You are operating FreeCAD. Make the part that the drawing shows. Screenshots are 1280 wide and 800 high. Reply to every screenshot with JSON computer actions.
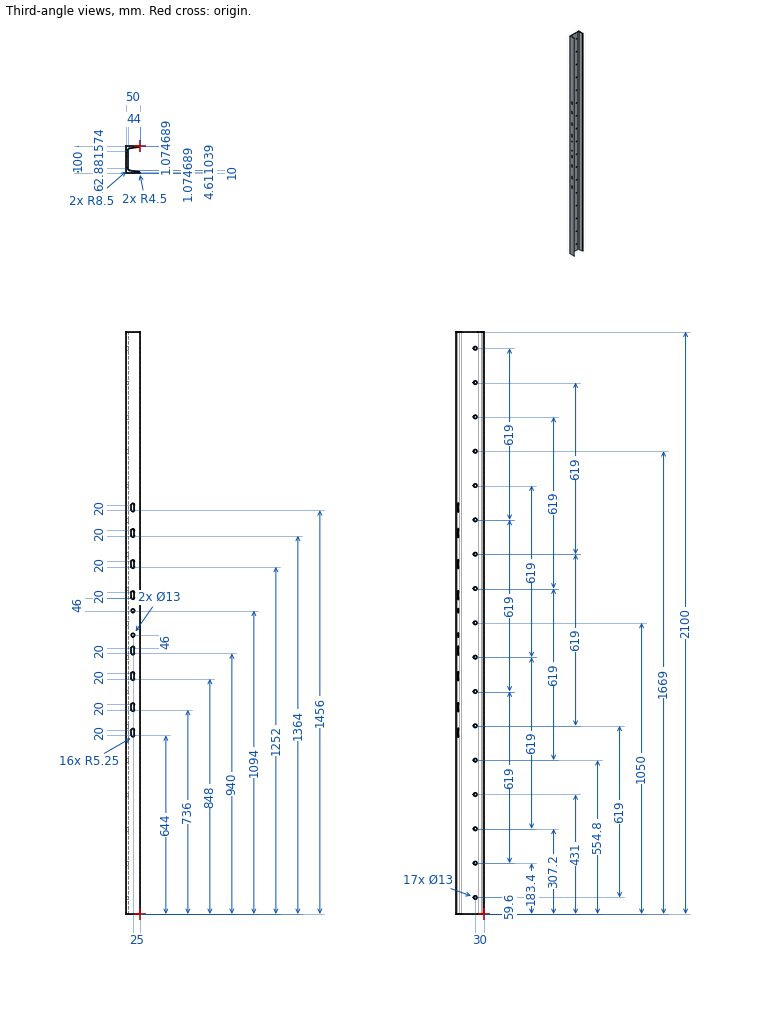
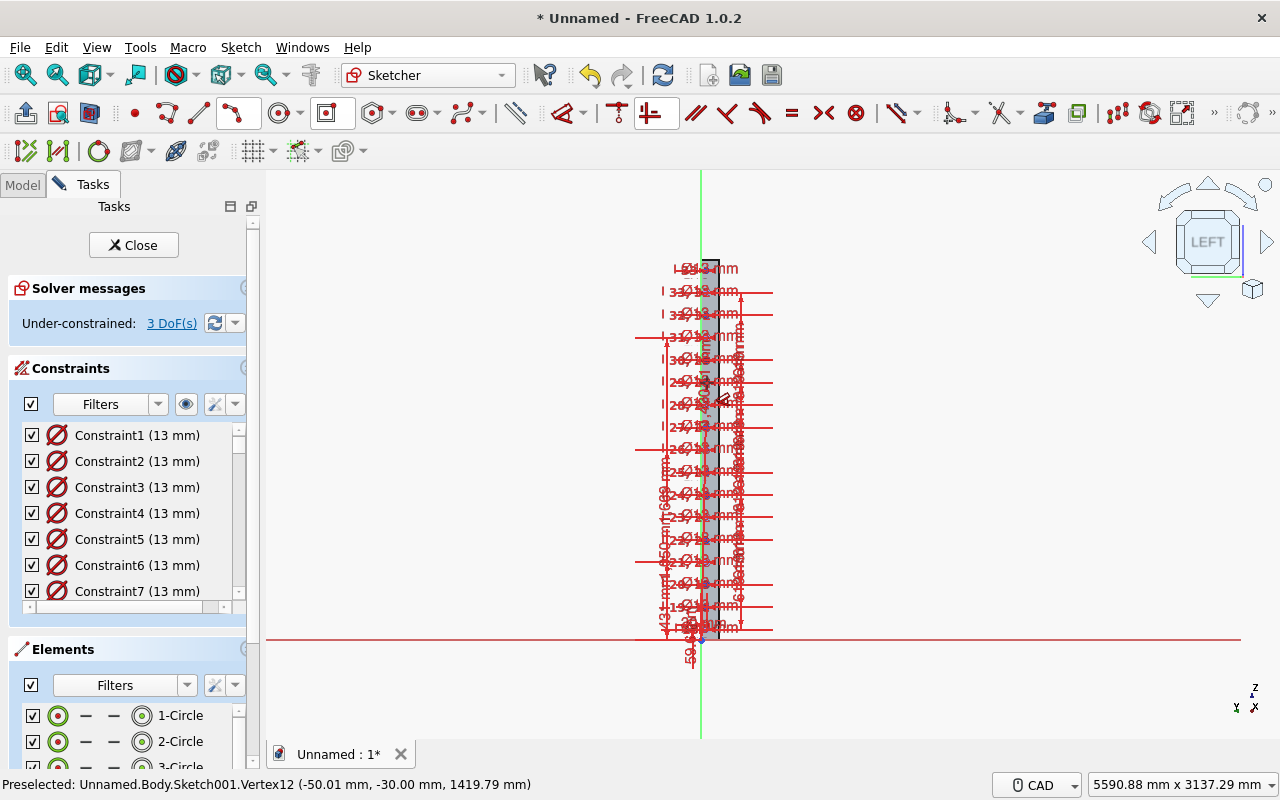
{"action": "left_click", "coordinate": [707, 271]}
{"action": "left_click", "coordinate": [741, 327]}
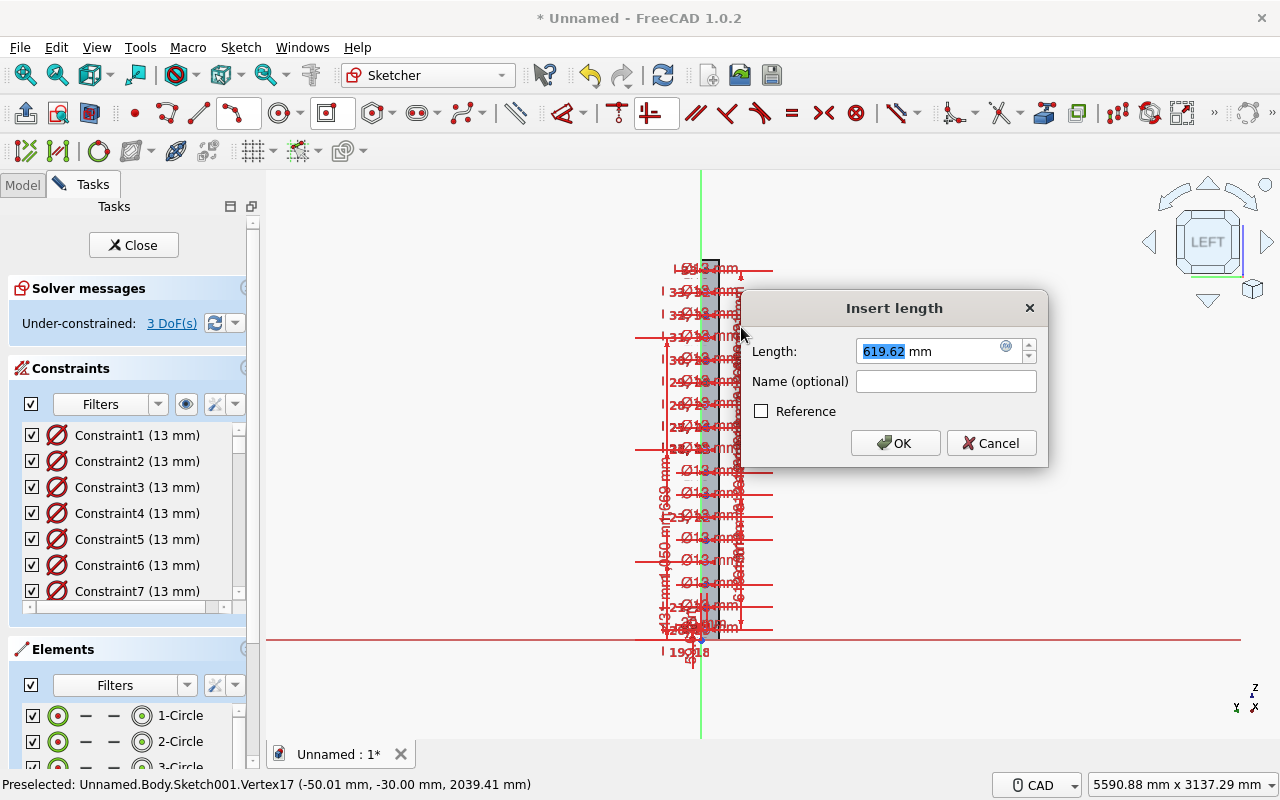
{"action": "type", "text": "619"}
{"action": "key", "text": "Return"}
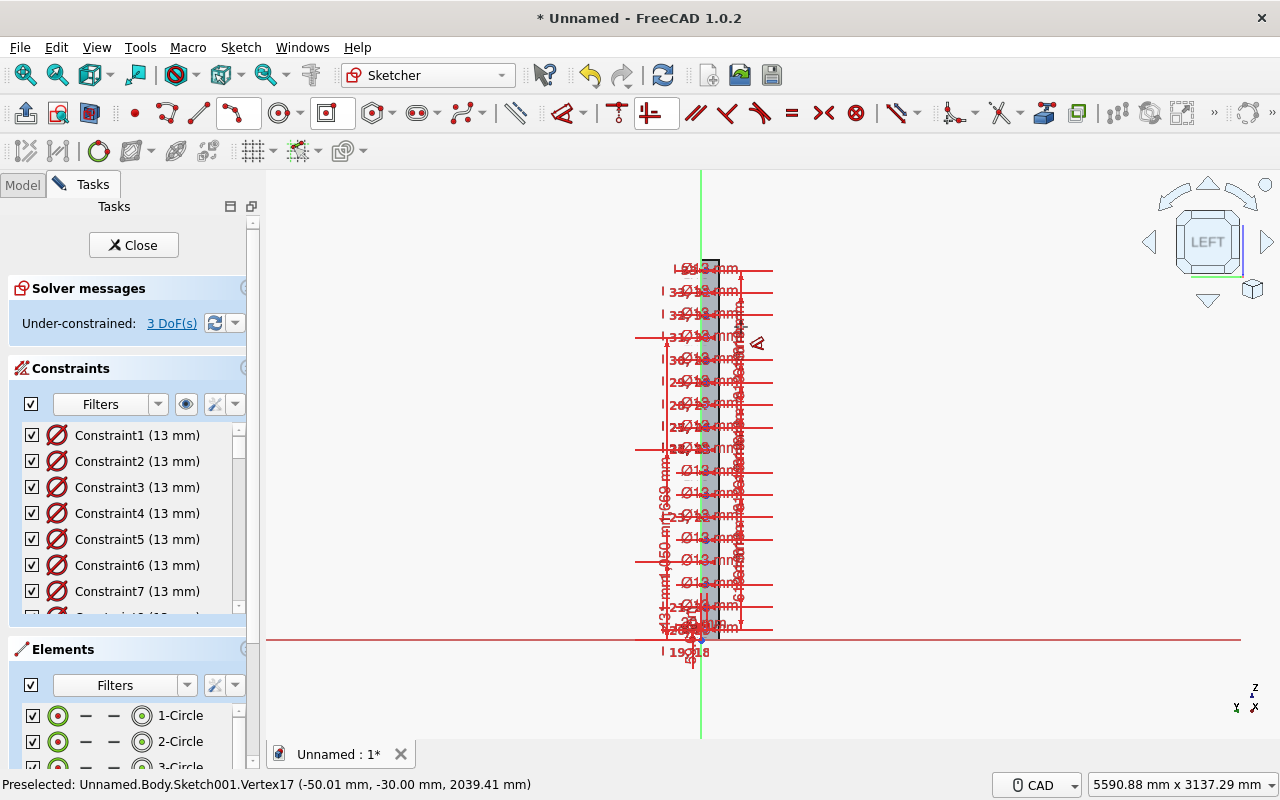
{"action": "left_click", "coordinate": [707, 607]}
{"action": "left_click", "coordinate": [619, 624]}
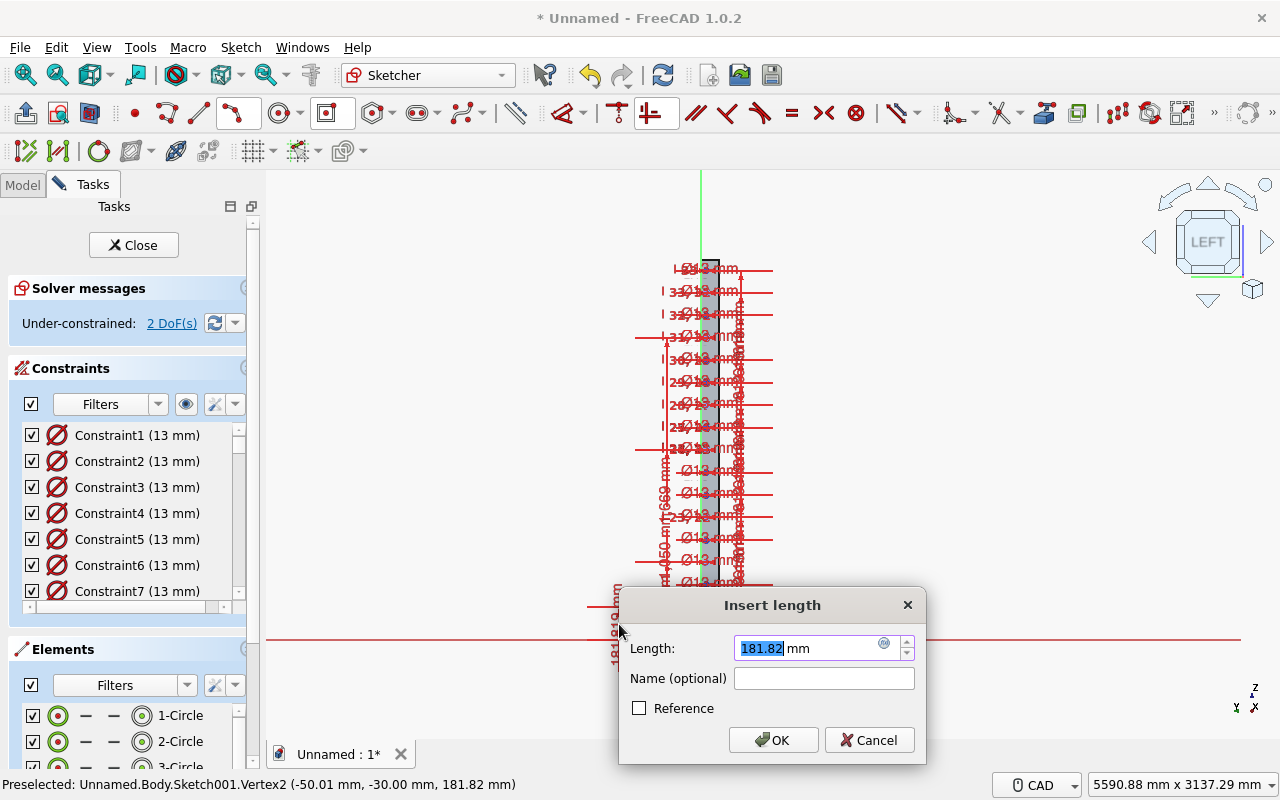
{"action": "type", "text": "183.4"}
{"action": "key", "text": "Return"}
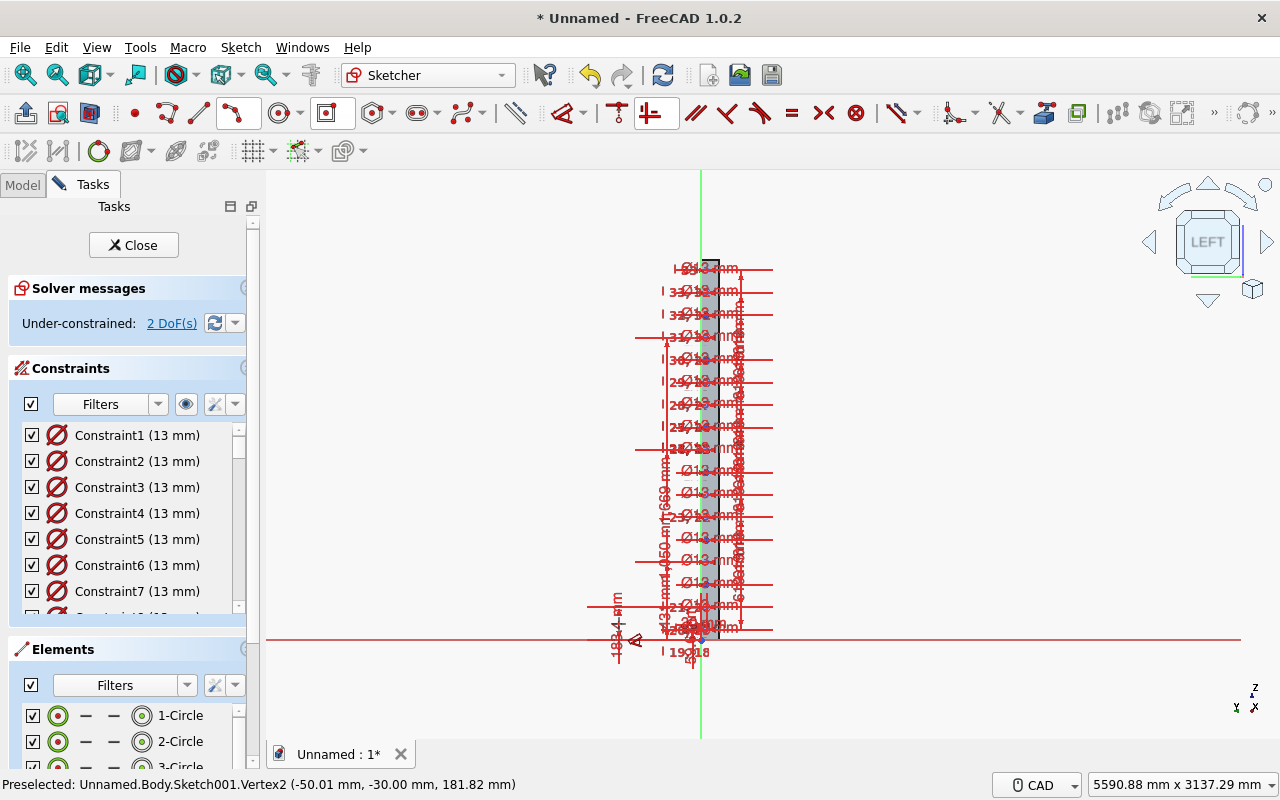
{"action": "left_click", "coordinate": [707, 585]}
{"action": "left_click", "coordinate": [741, 600]}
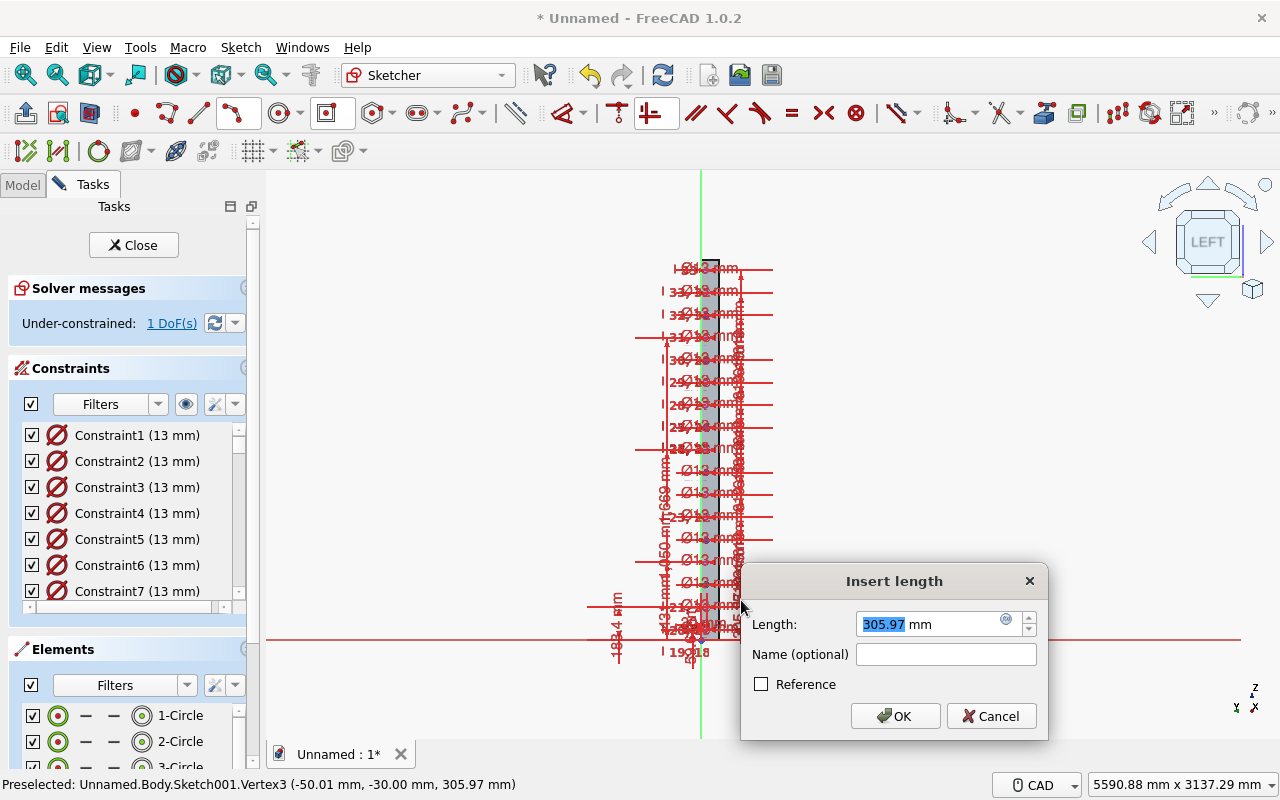
{"action": "type", "text": "307.2"}
{"action": "key", "text": "Return"}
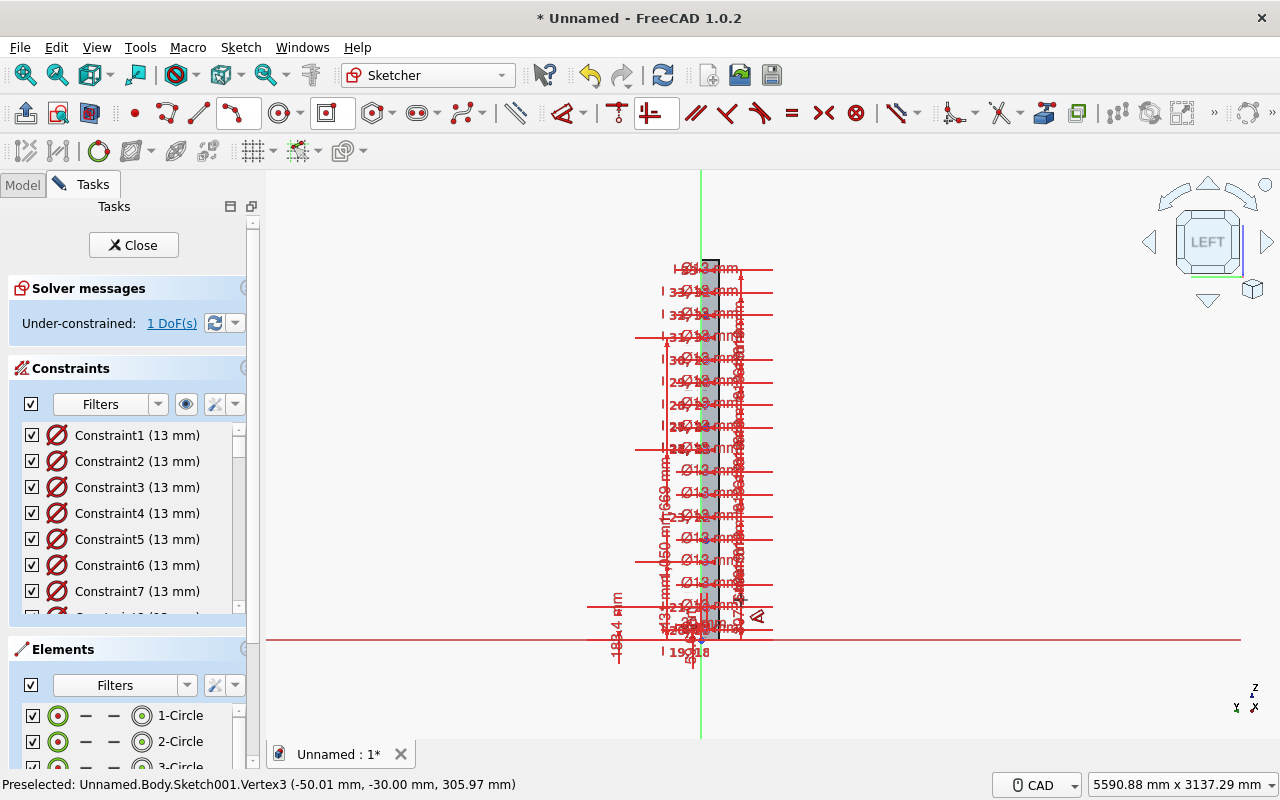
{"action": "left_click", "coordinate": [707, 540]}
{"action": "left_click", "coordinate": [667, 567]}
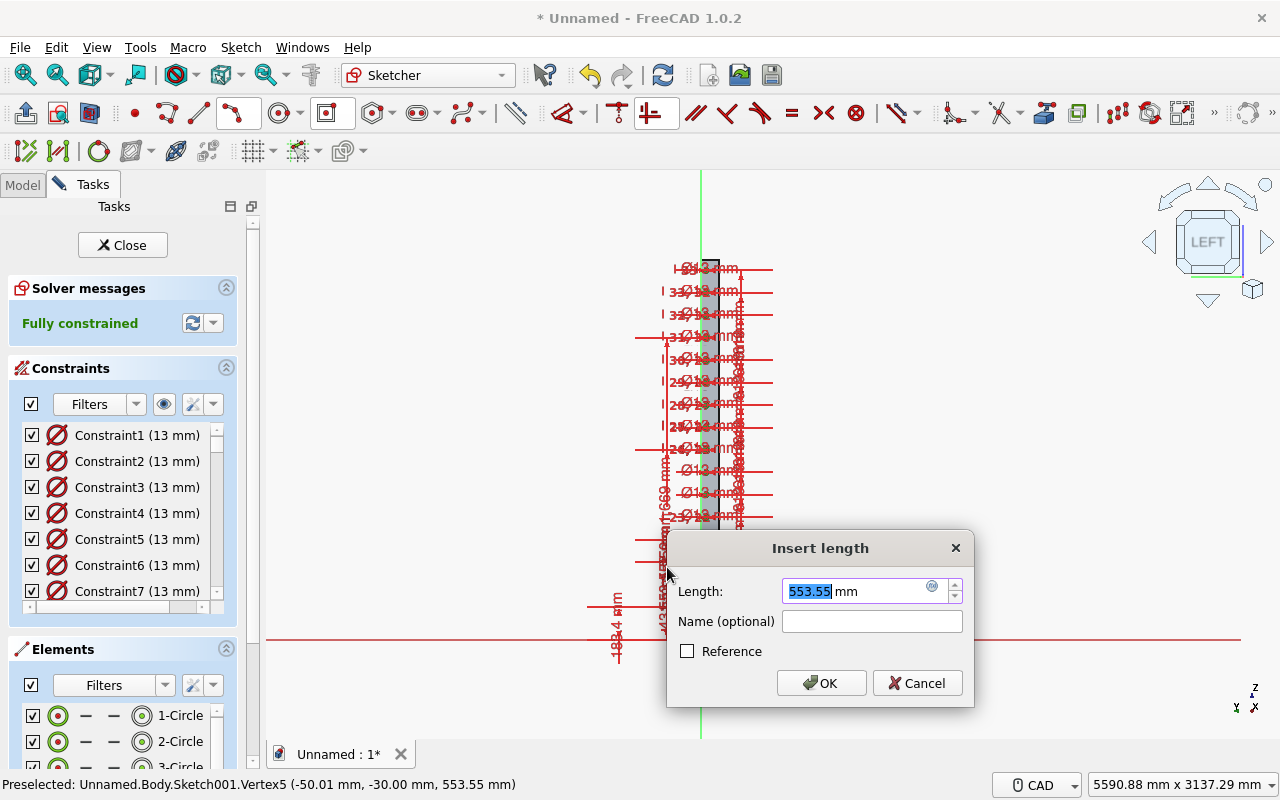
{"action": "type", "text": "554.8"}
{"action": "key", "text": "Return"}
{"action": "key", "text": "Escape"}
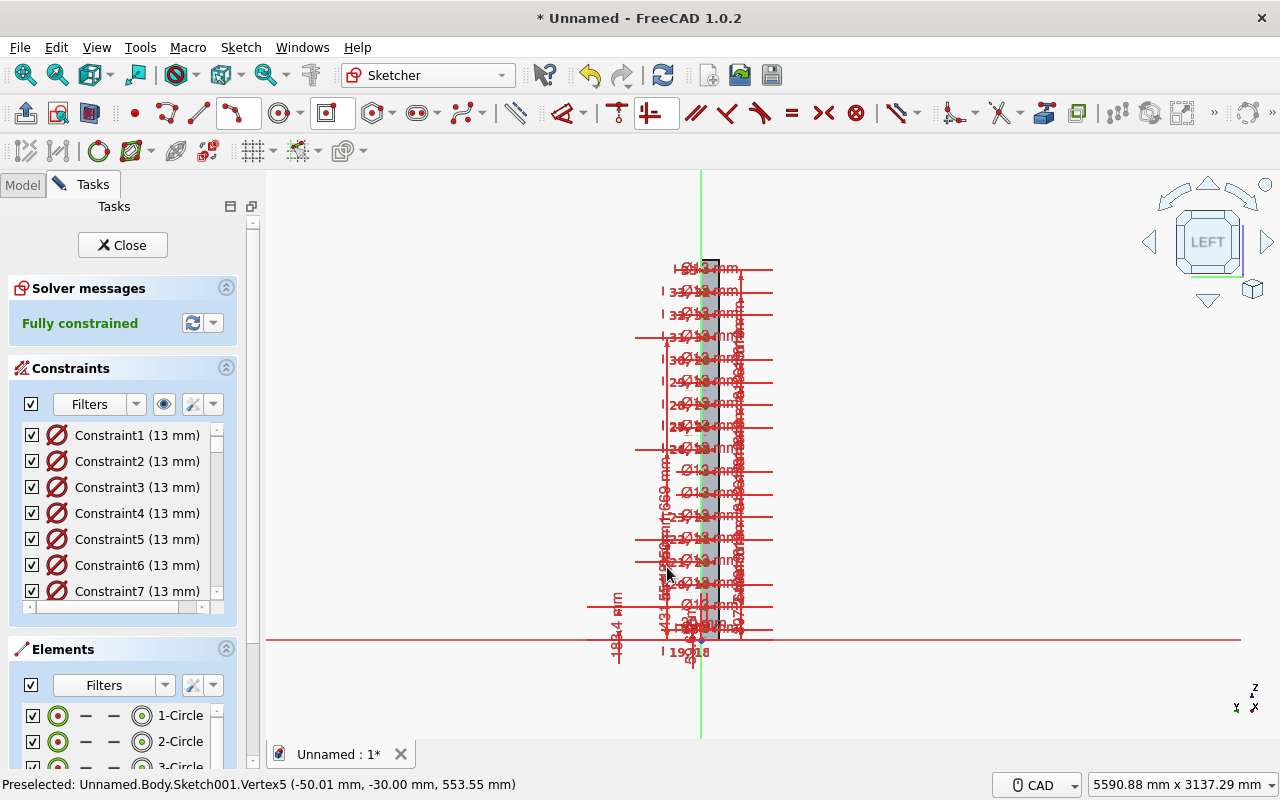
{"action": "left_click", "coordinate": [123, 245]}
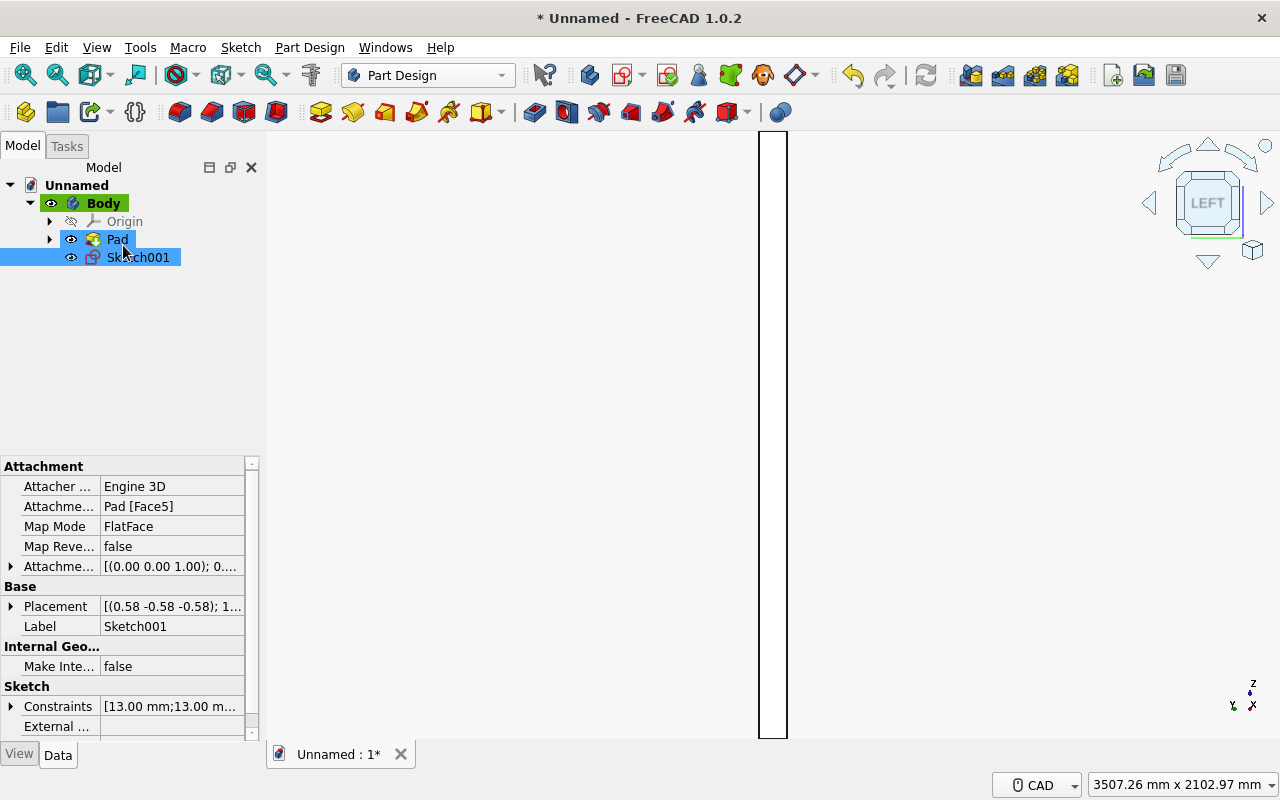
{"action": "left_click", "coordinate": [536, 112]}